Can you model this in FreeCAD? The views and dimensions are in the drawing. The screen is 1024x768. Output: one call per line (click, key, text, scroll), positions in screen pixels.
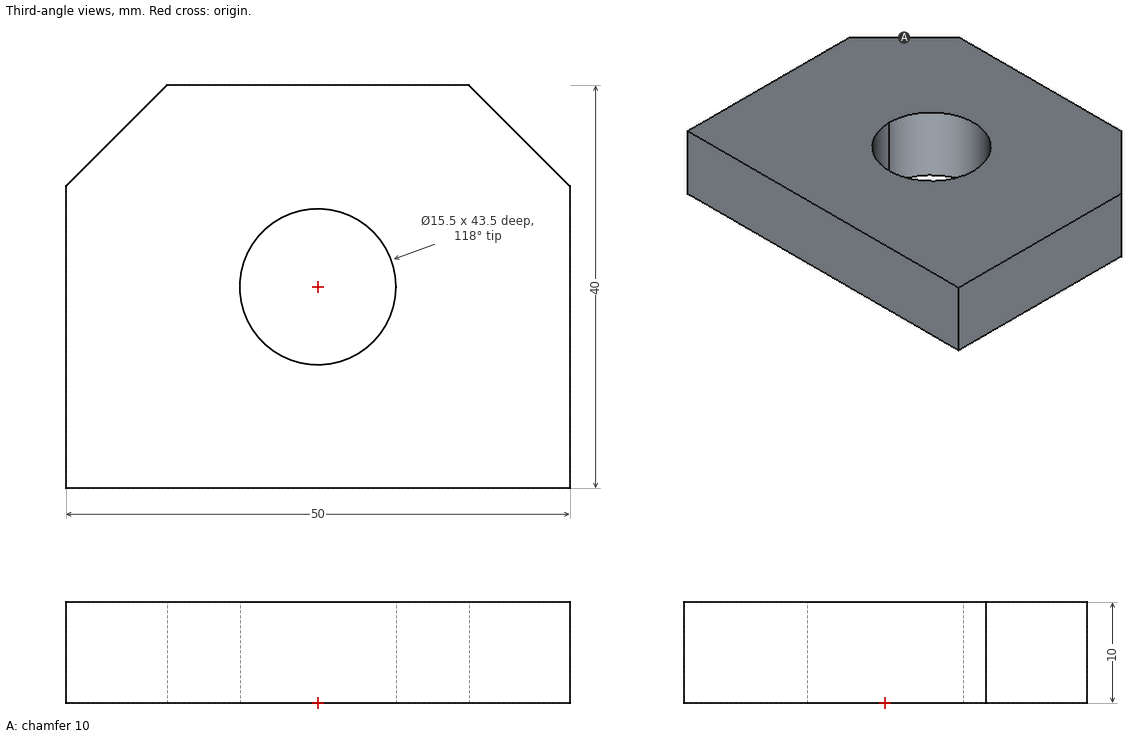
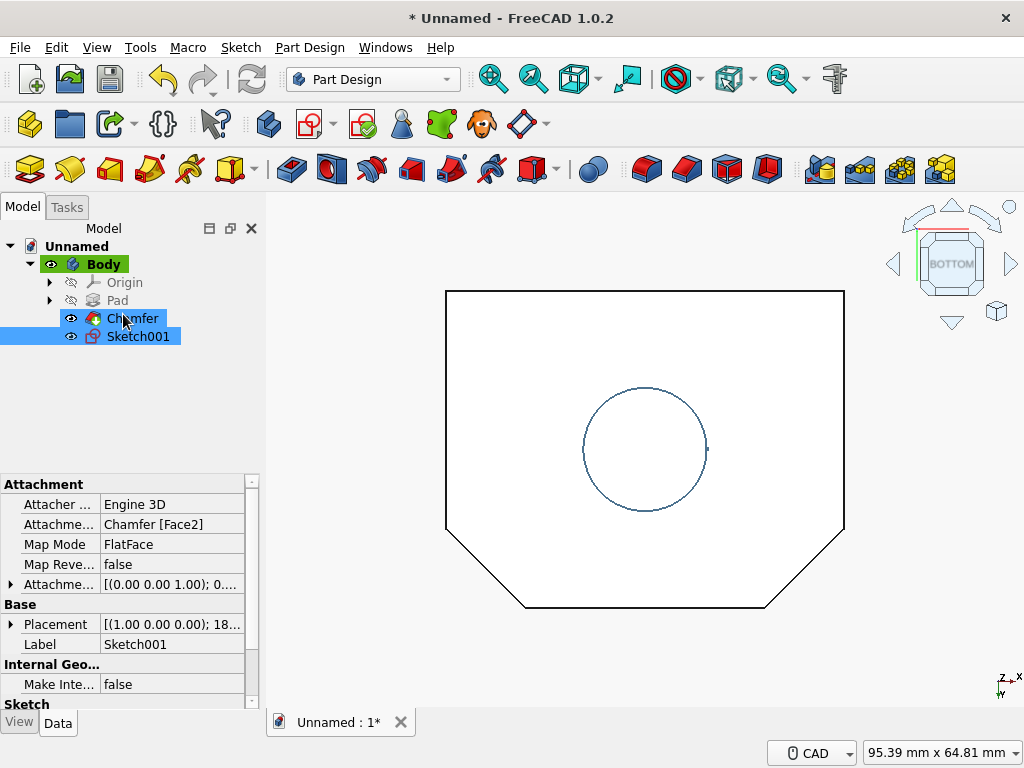
click(332, 170)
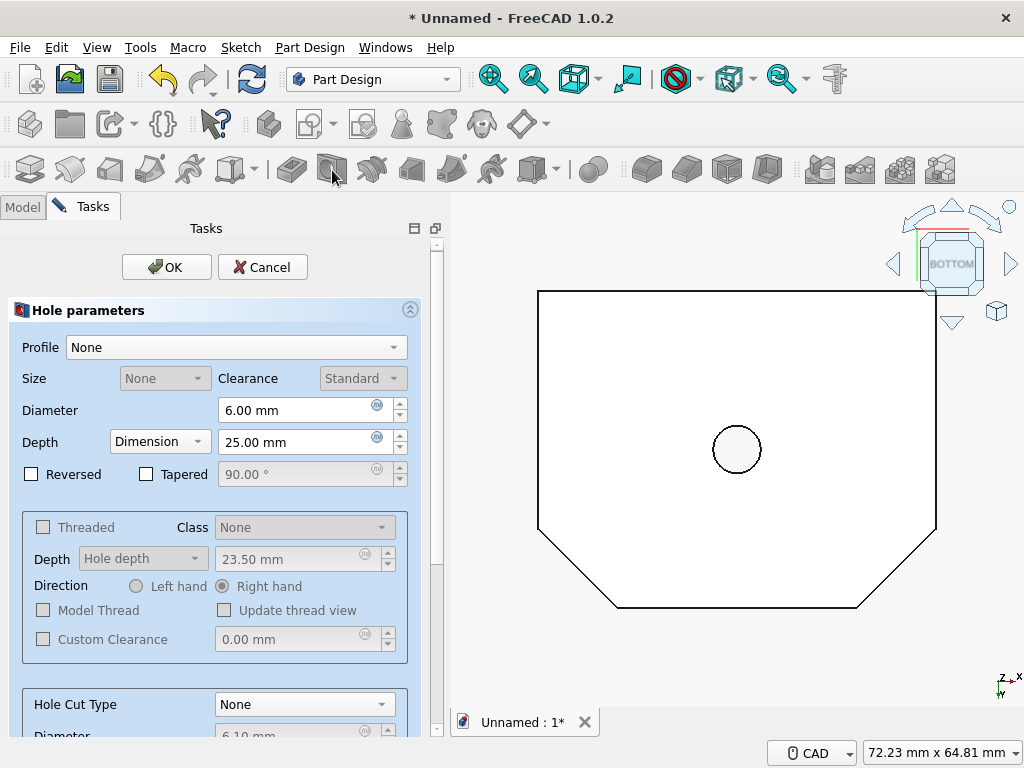
triple_click(305, 410)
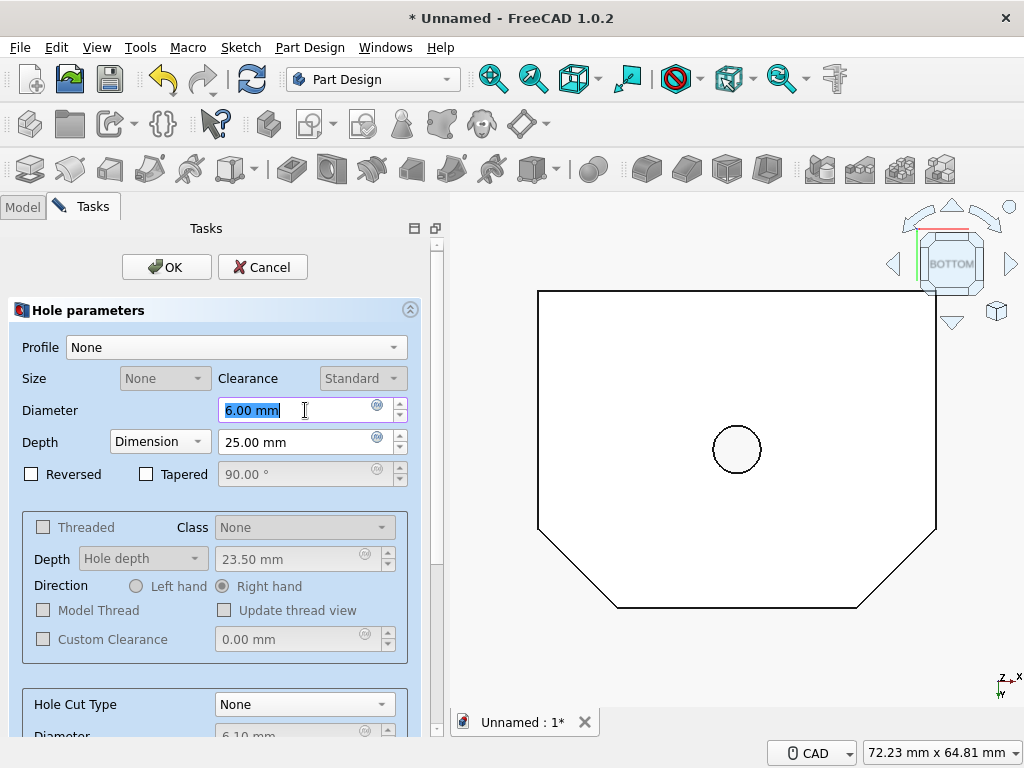
text(15.5)
key(Tab)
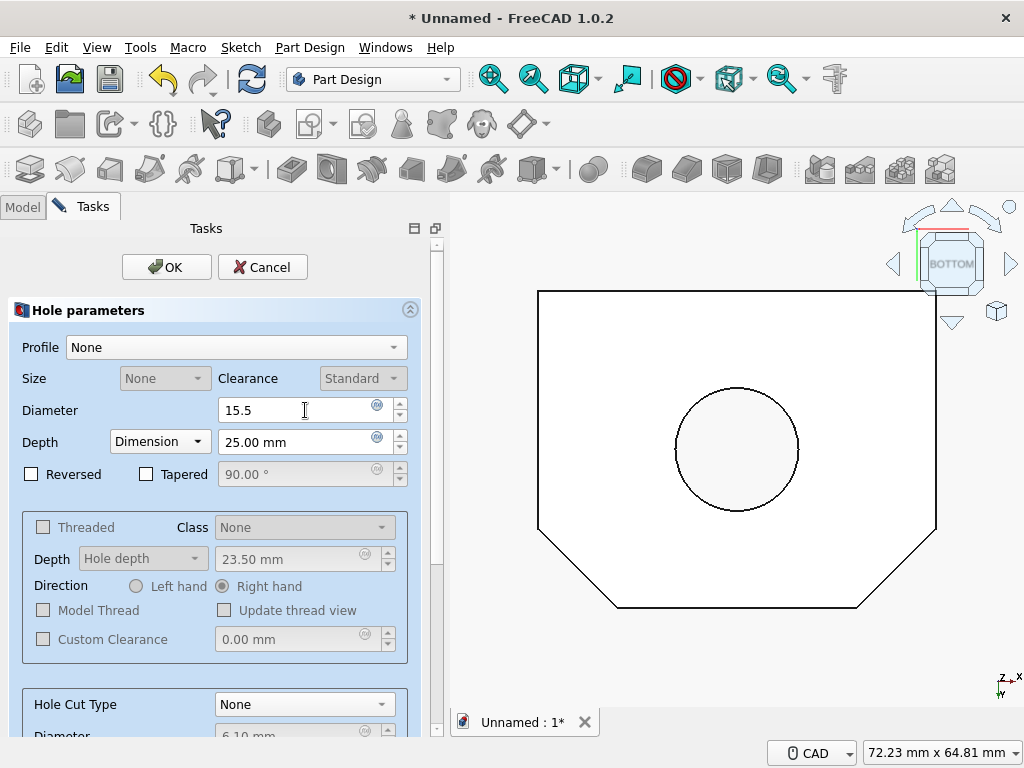
triple_click(305, 442)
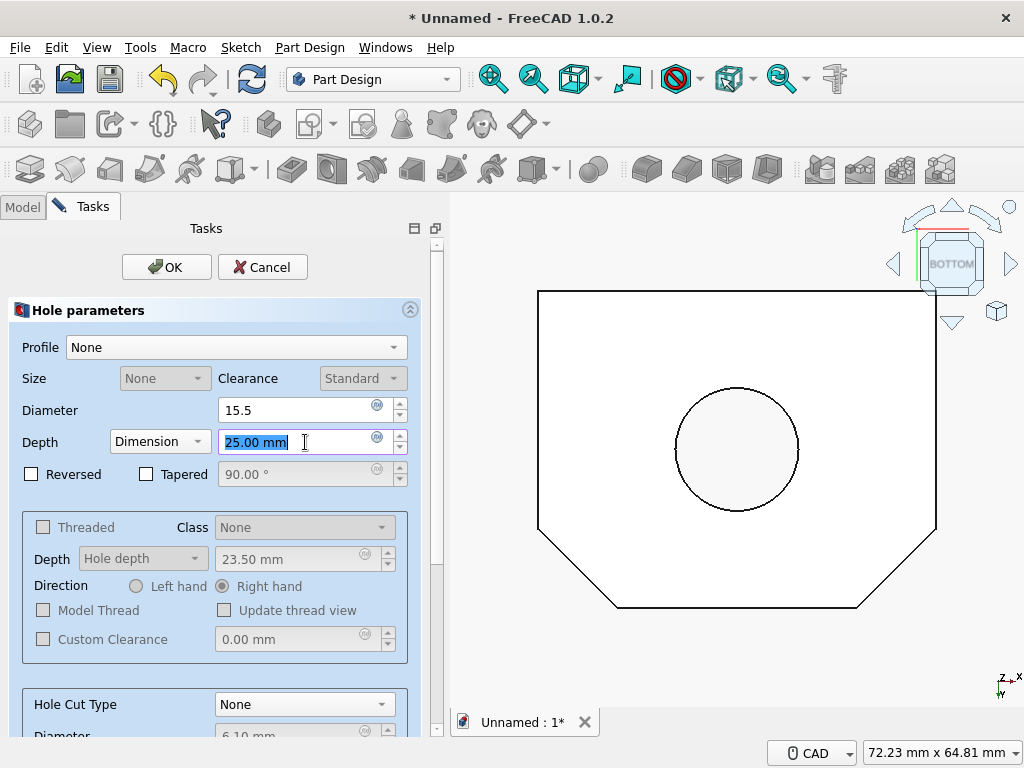
text(43.5)
key(Tab)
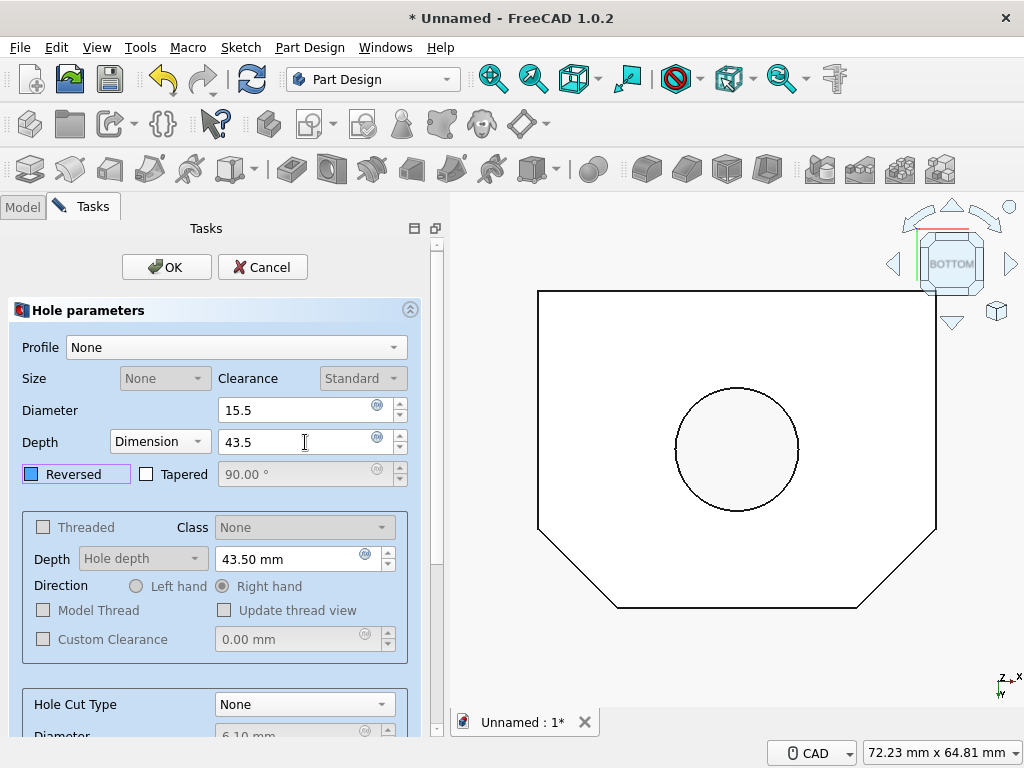
click(167, 267)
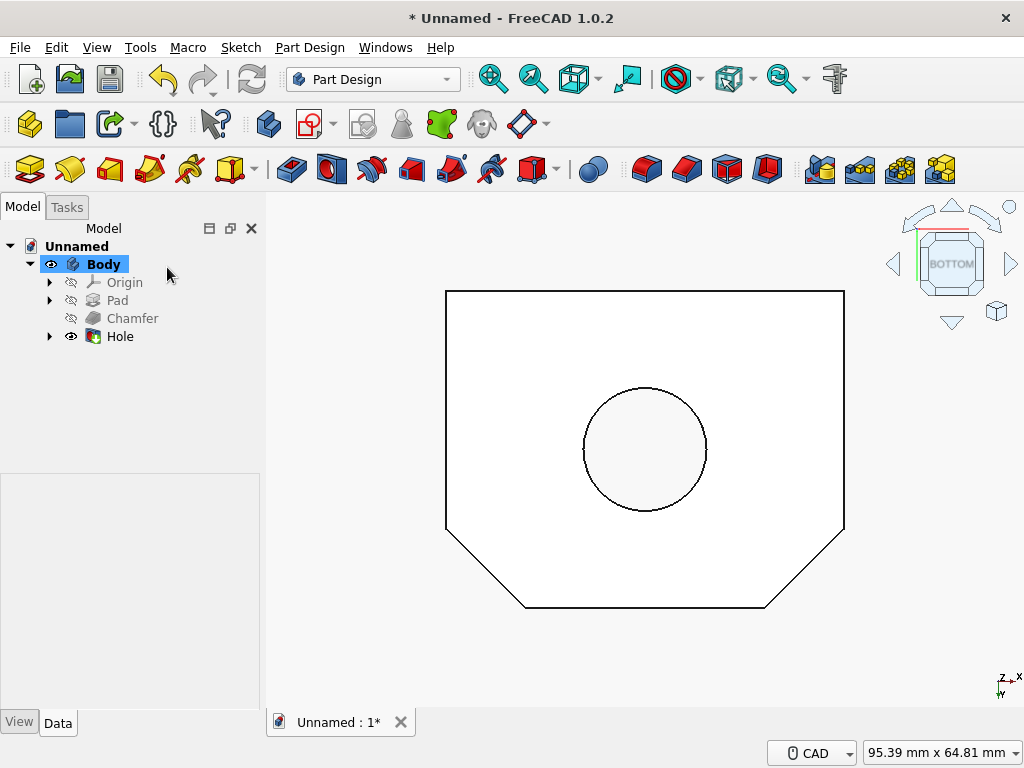
key(0)